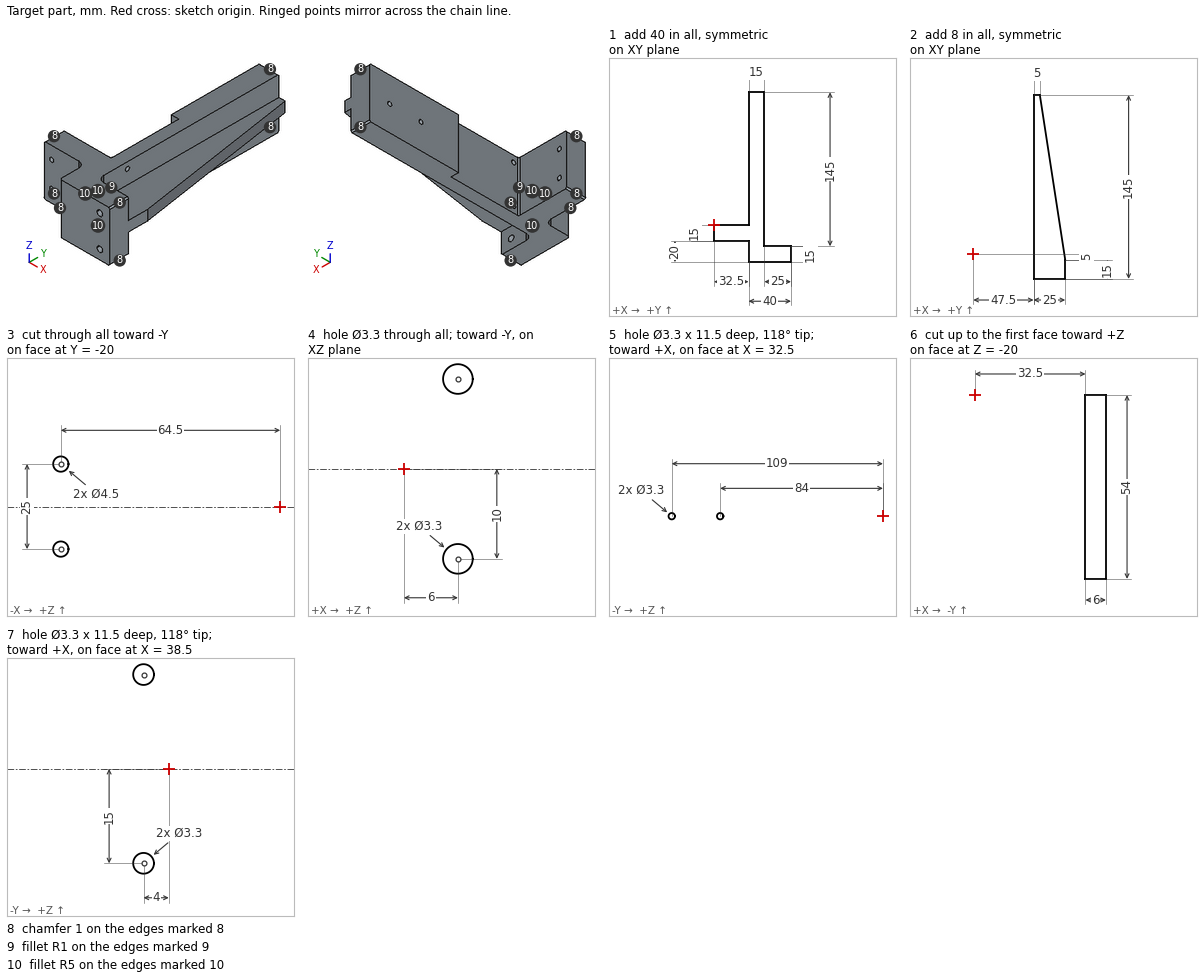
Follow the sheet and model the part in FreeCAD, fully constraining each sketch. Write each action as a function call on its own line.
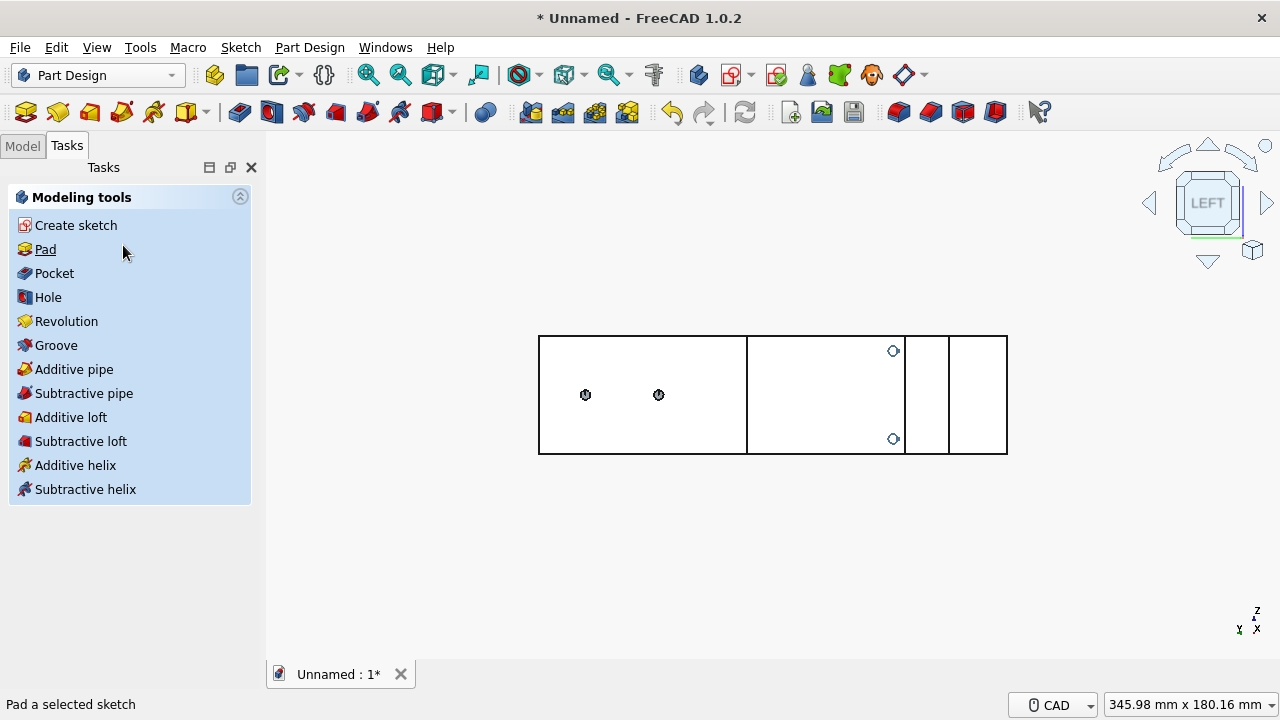
click(272, 112)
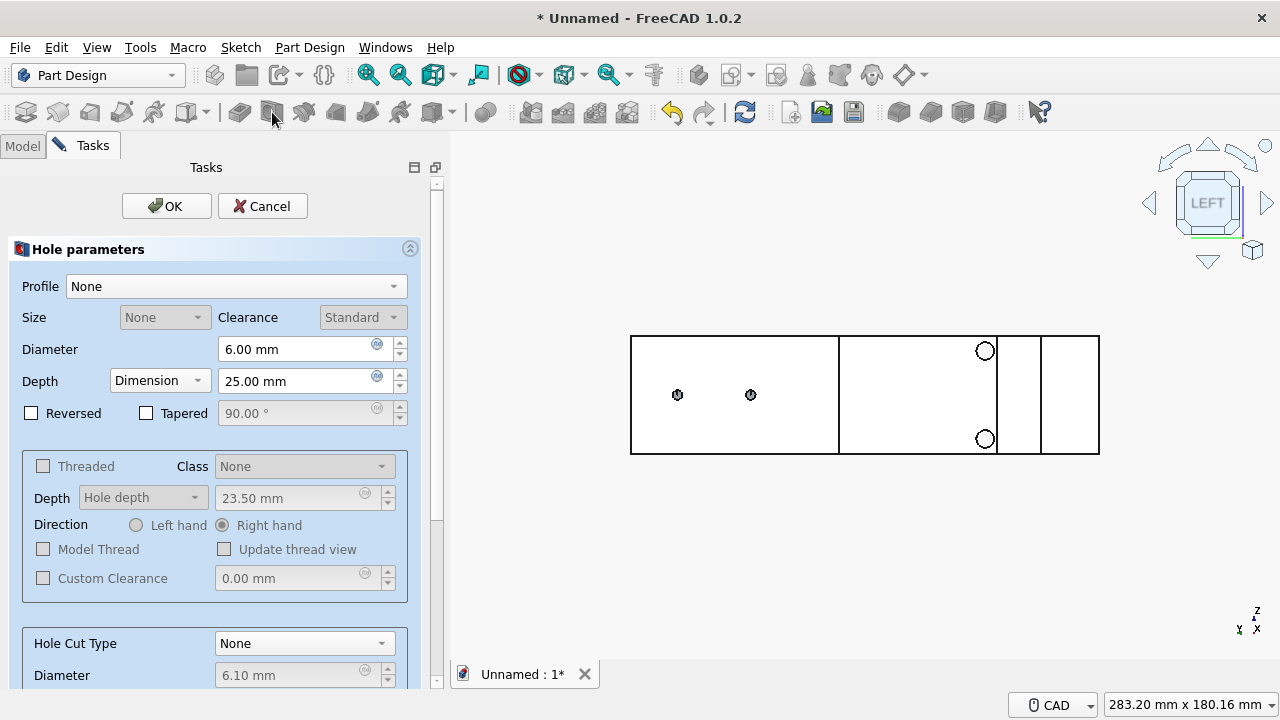
triple_click(305, 349)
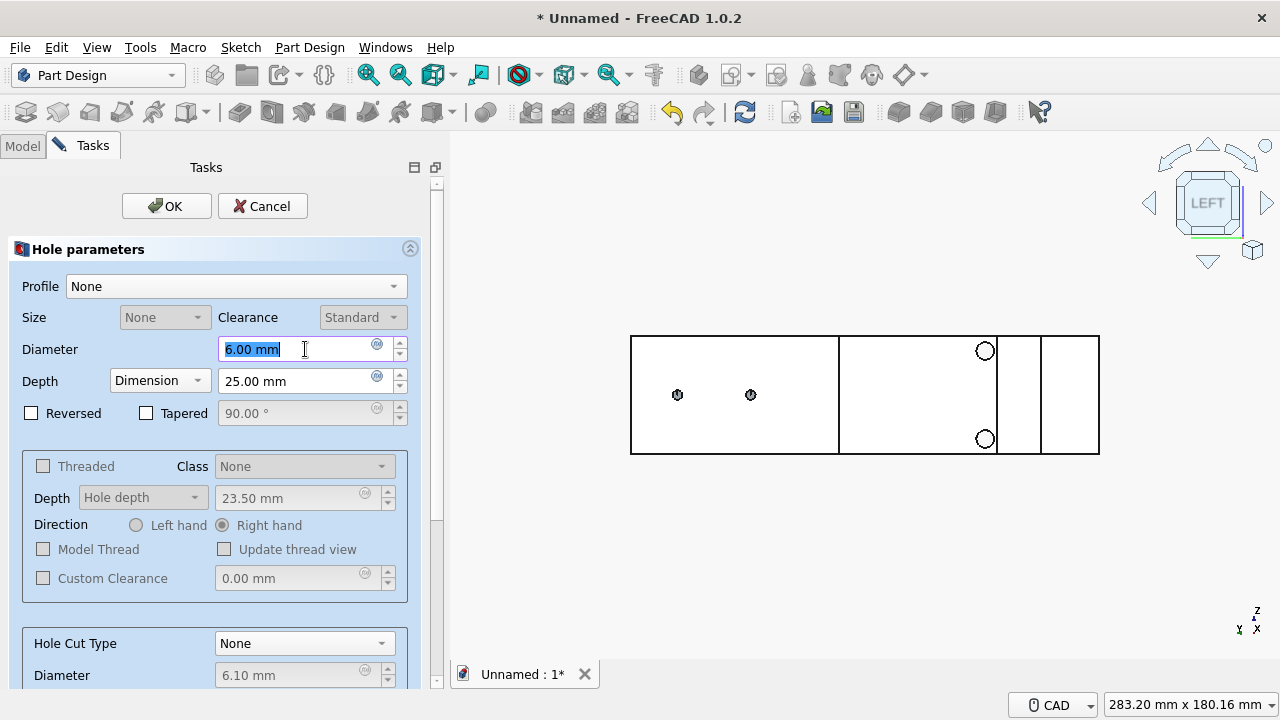
text(3.3)
key(Tab)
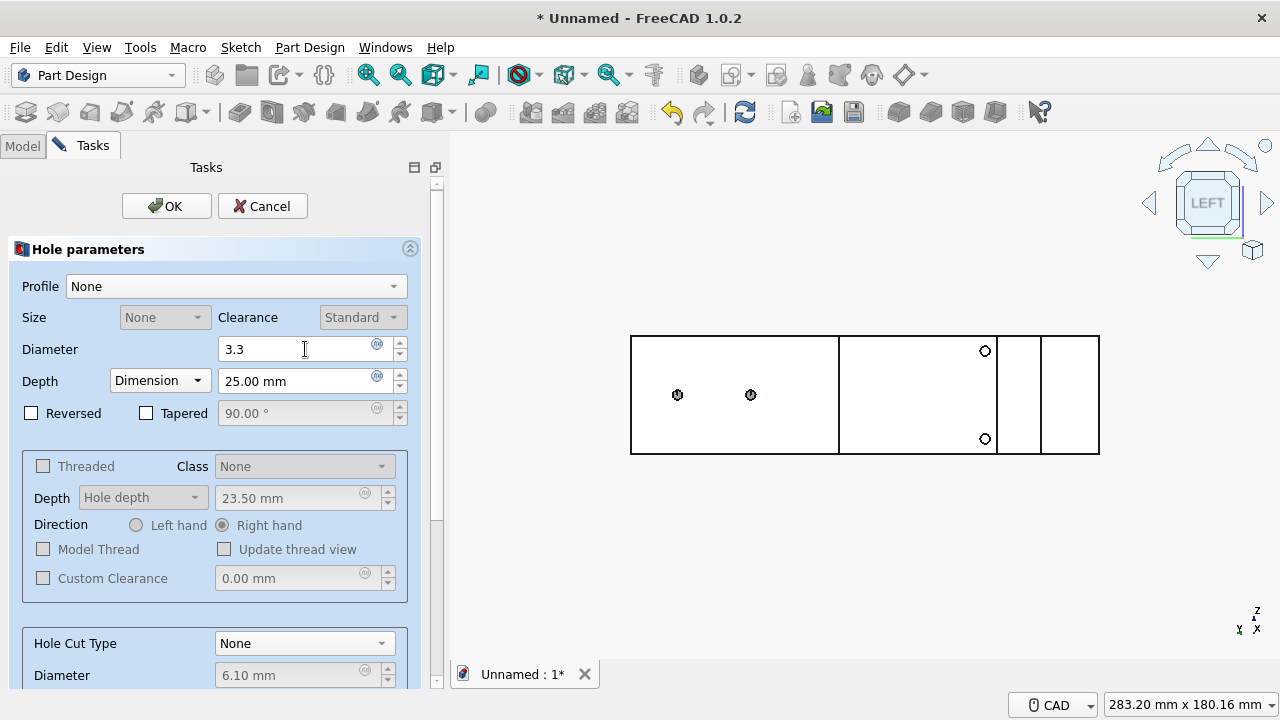
triple_click(305, 381)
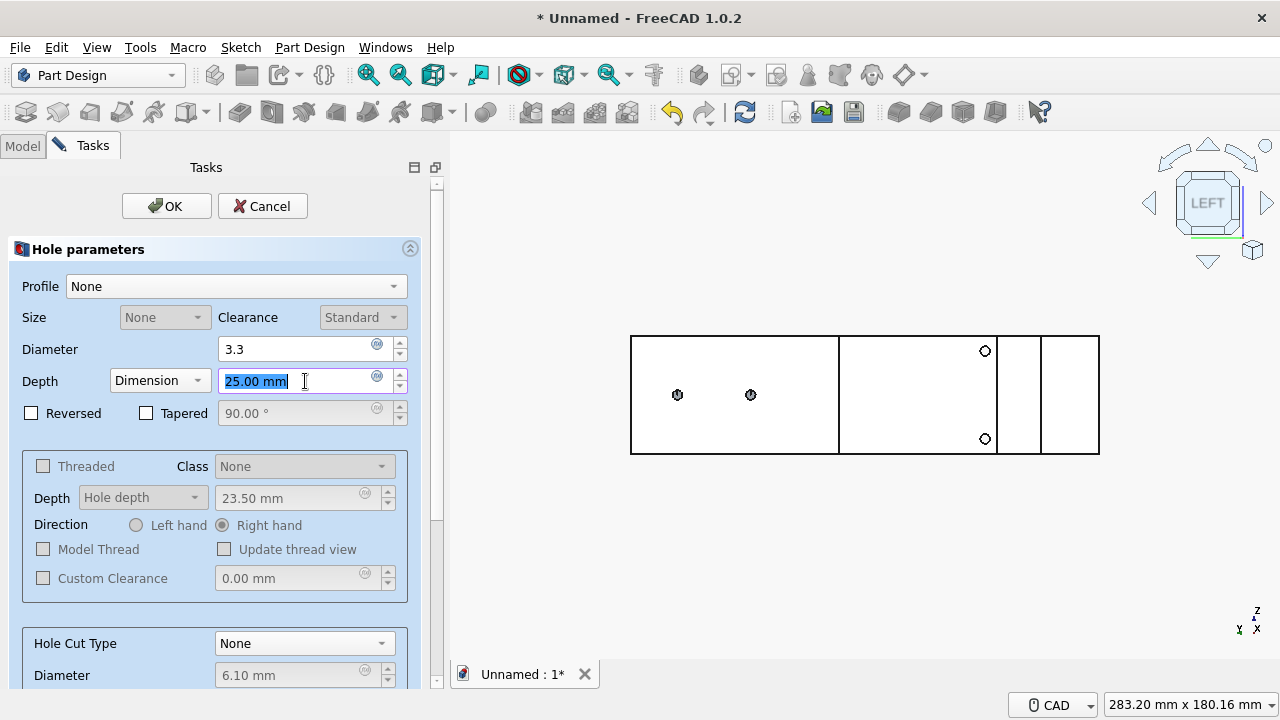
text(11.5)
key(Tab)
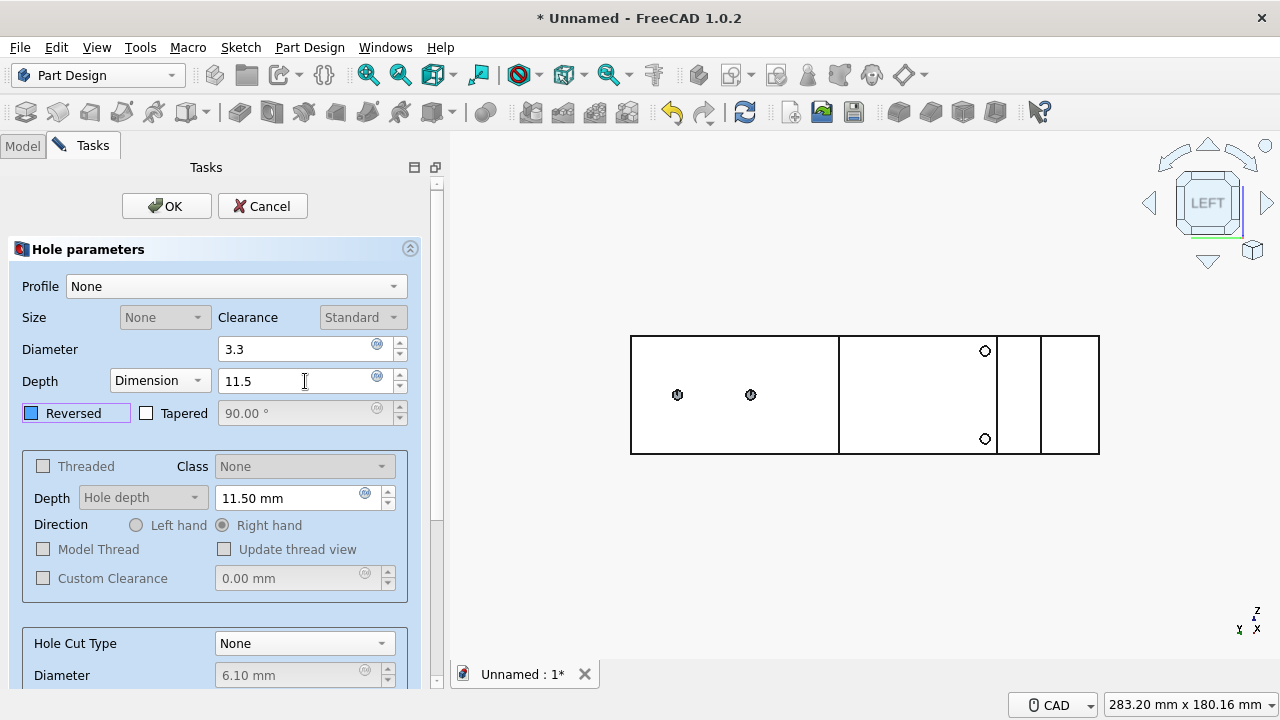
click(167, 206)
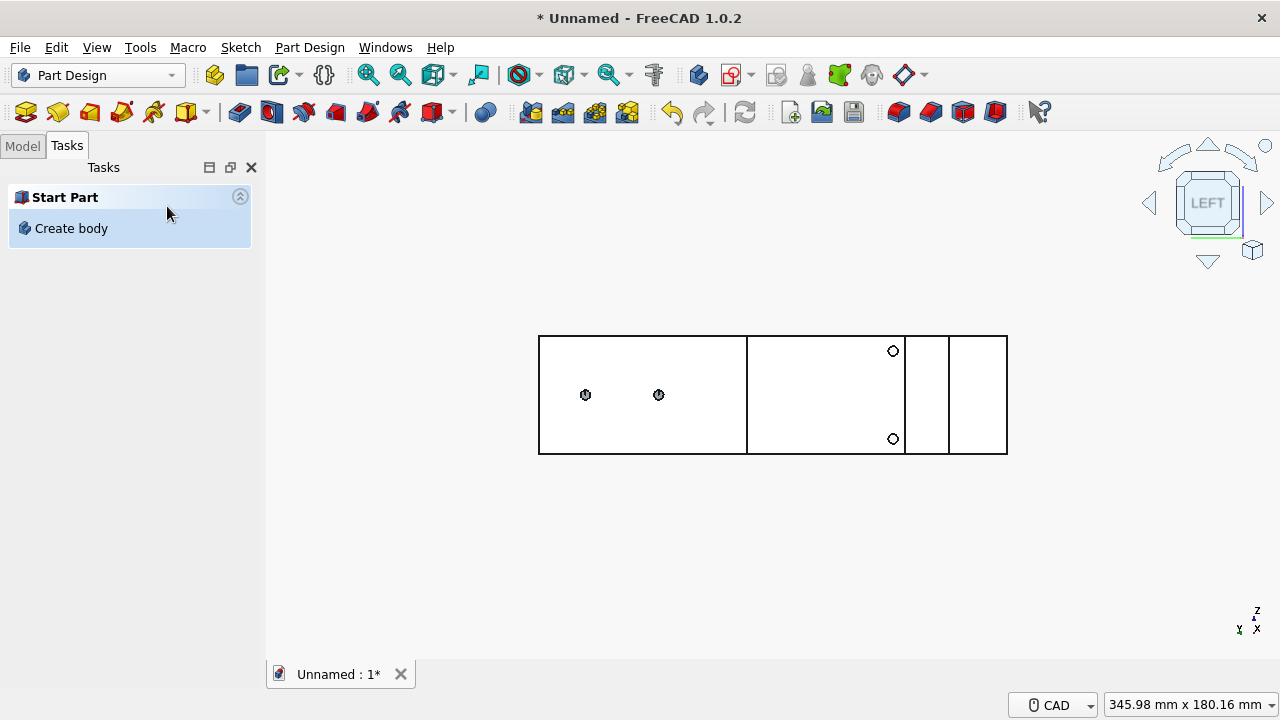
click(927, 453)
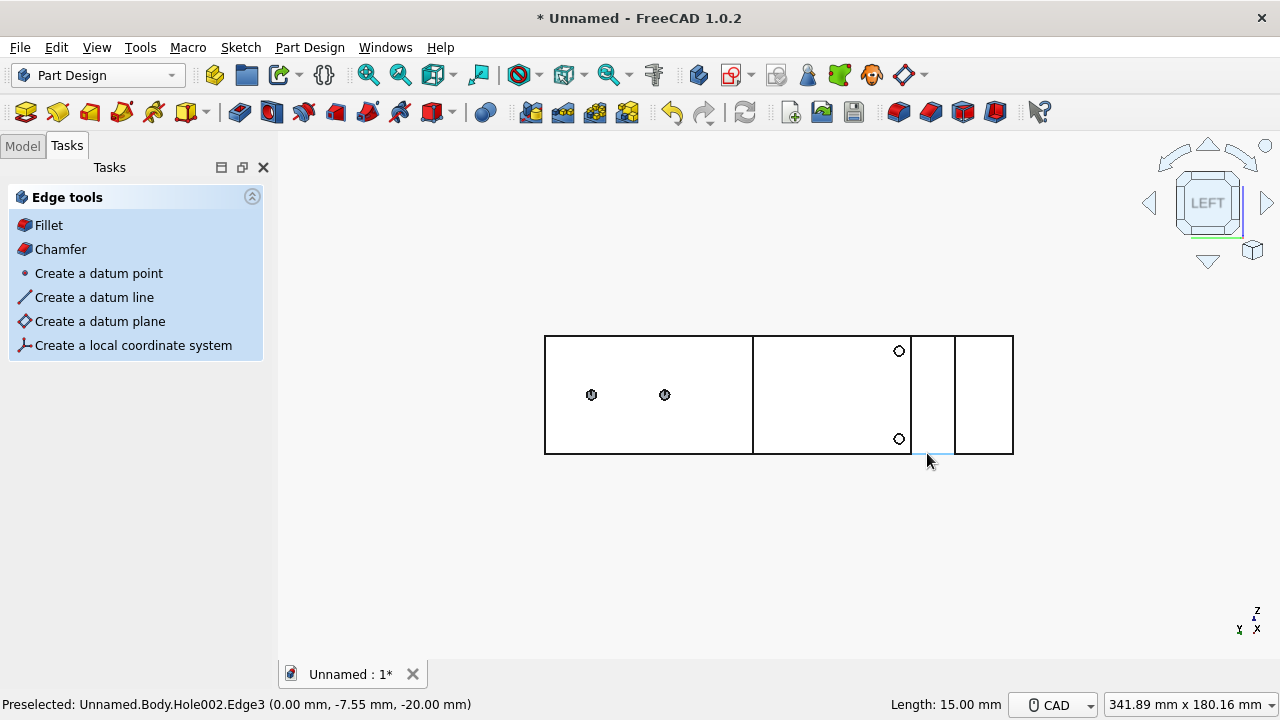
click(1013, 394, ctrl)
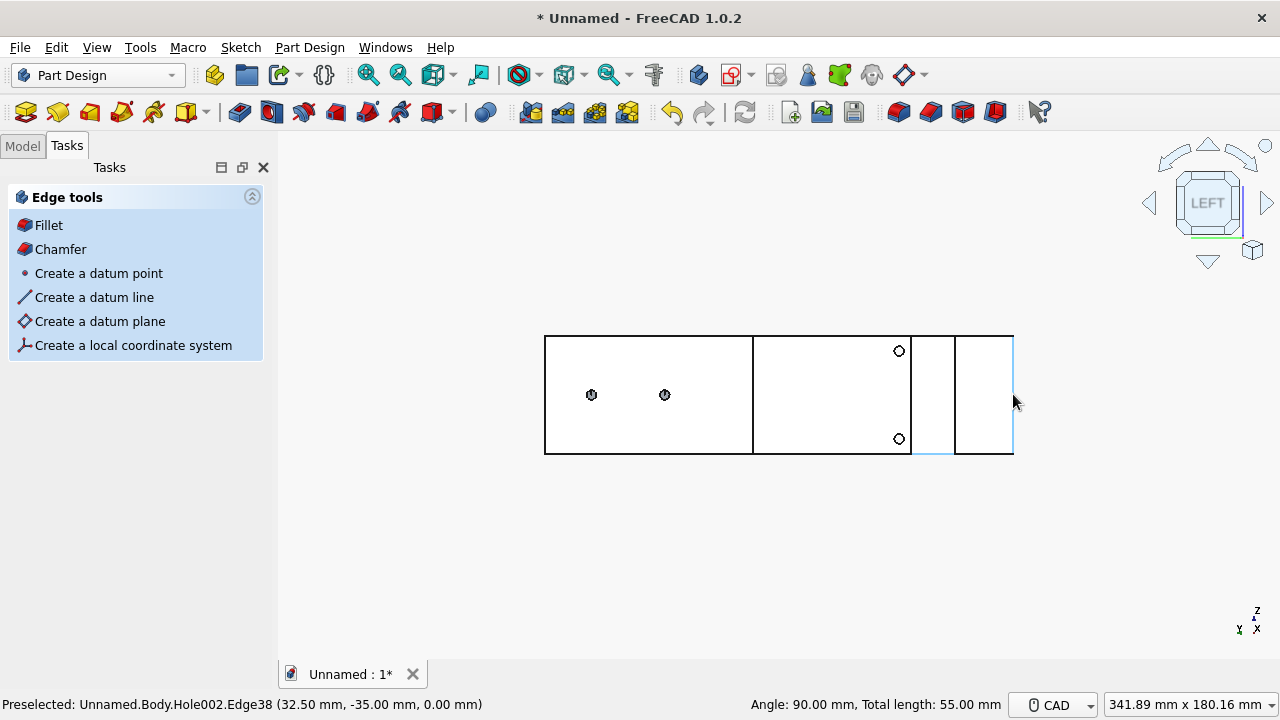
click(933, 335, ctrl)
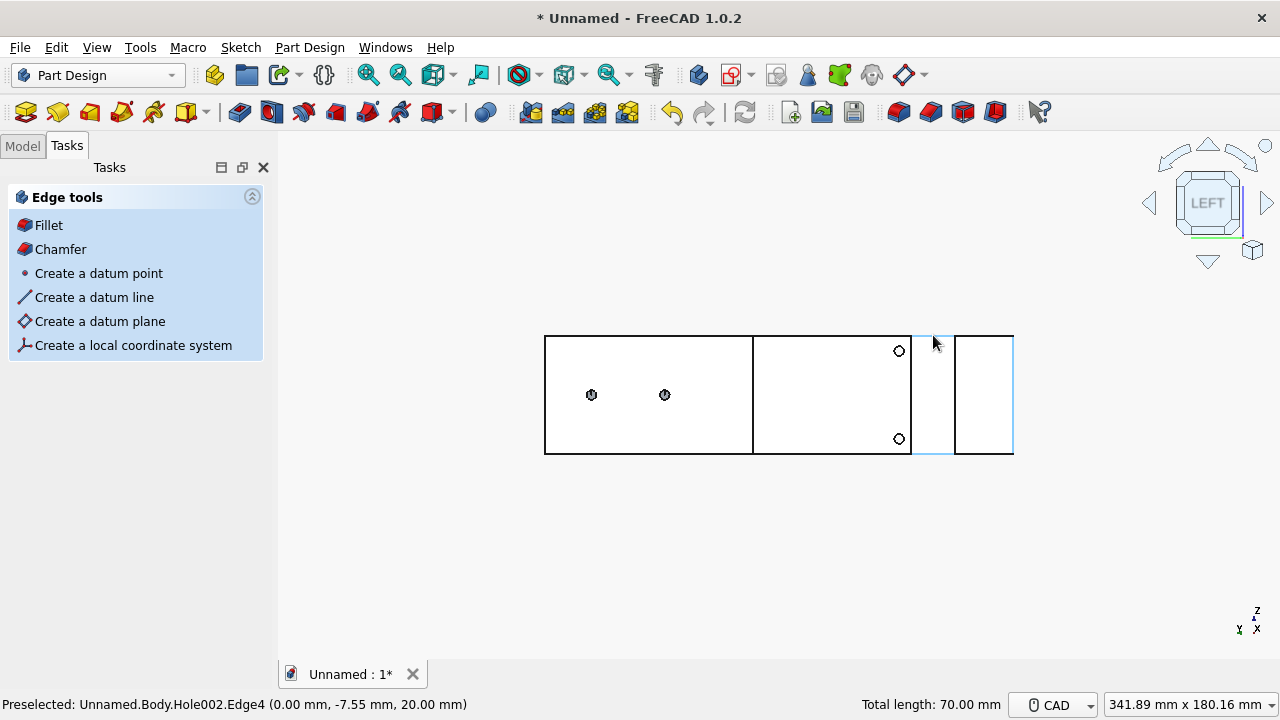
key(0)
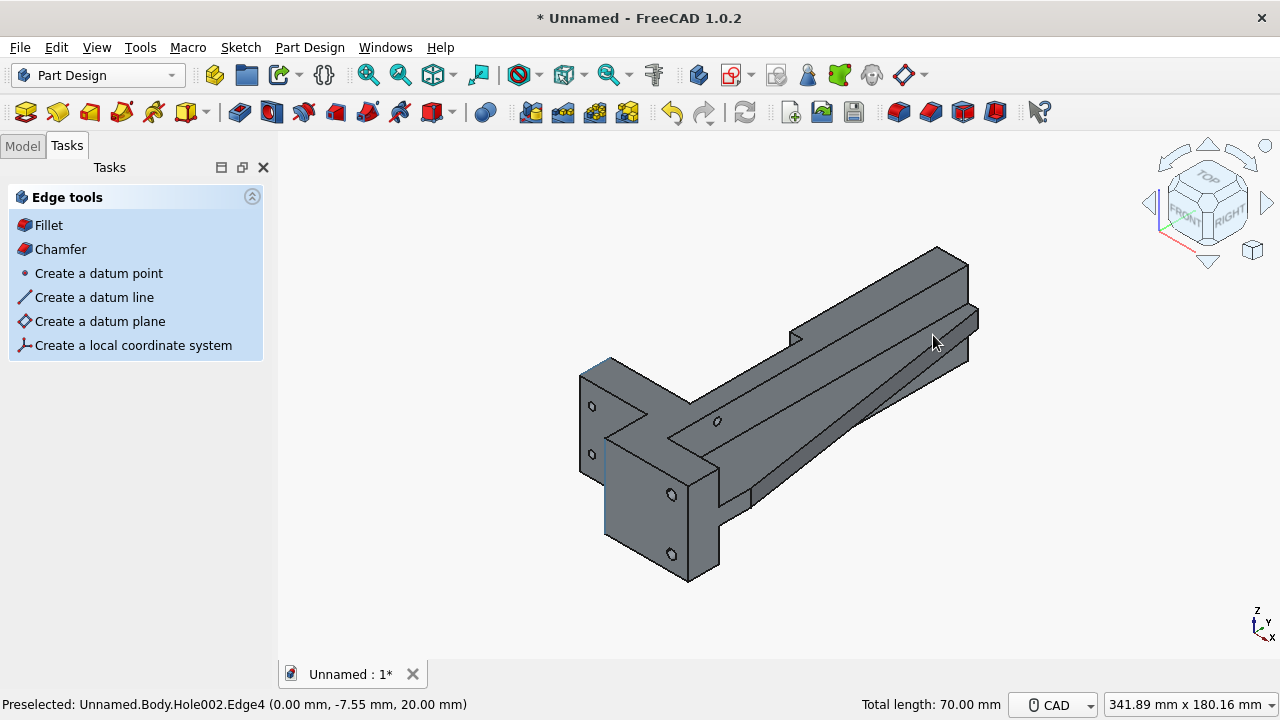
click(704, 476, ctrl)